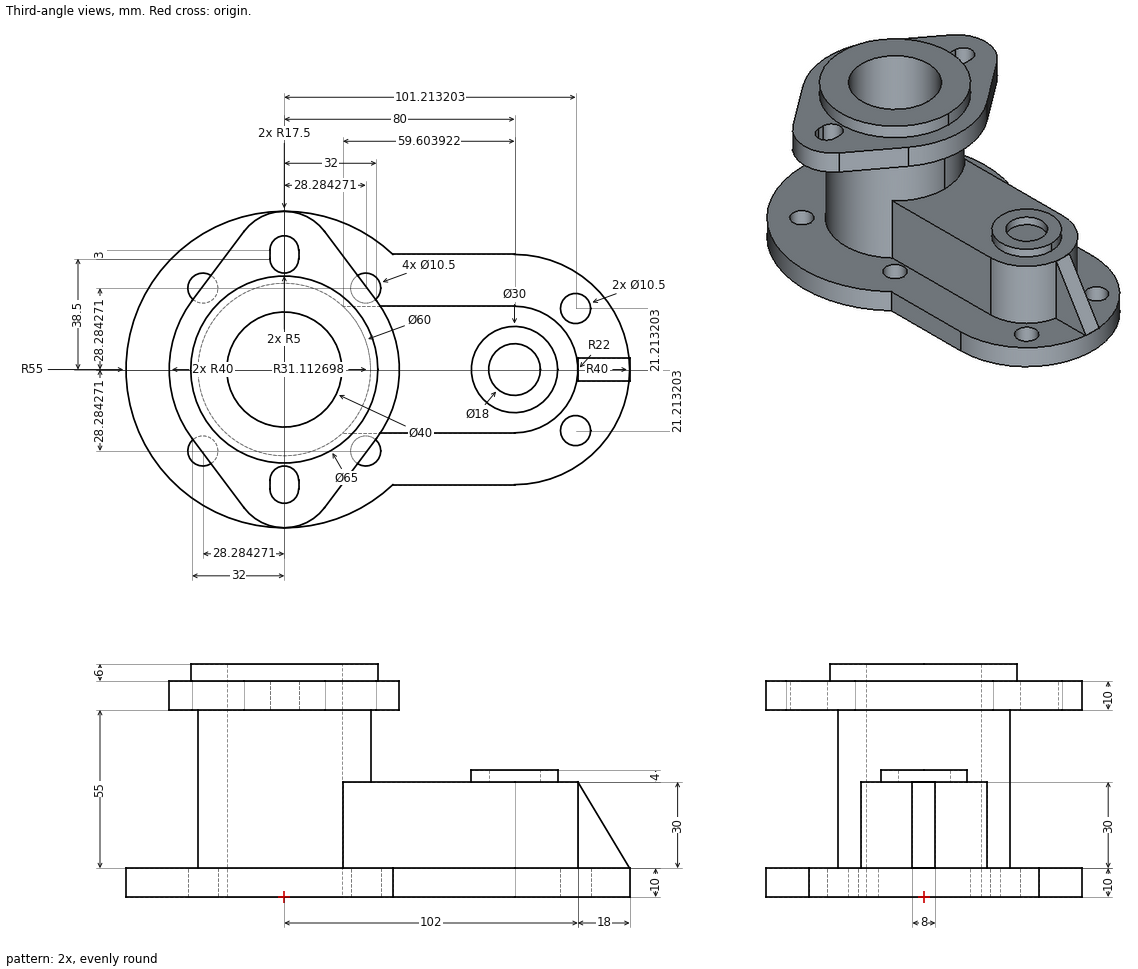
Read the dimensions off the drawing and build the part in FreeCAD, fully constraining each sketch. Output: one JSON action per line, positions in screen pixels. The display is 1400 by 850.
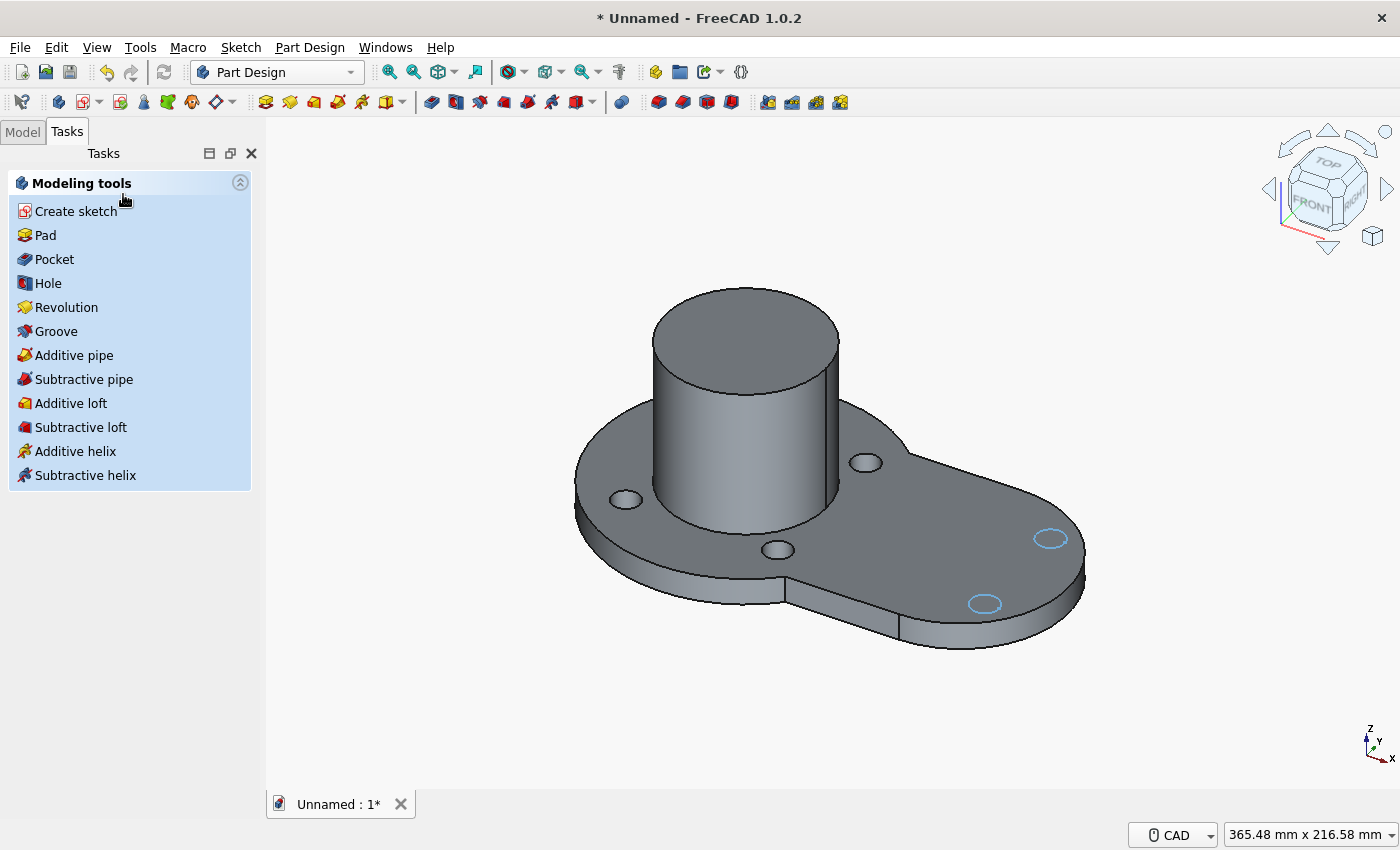
{"action": "left_click", "coordinate": [432, 102]}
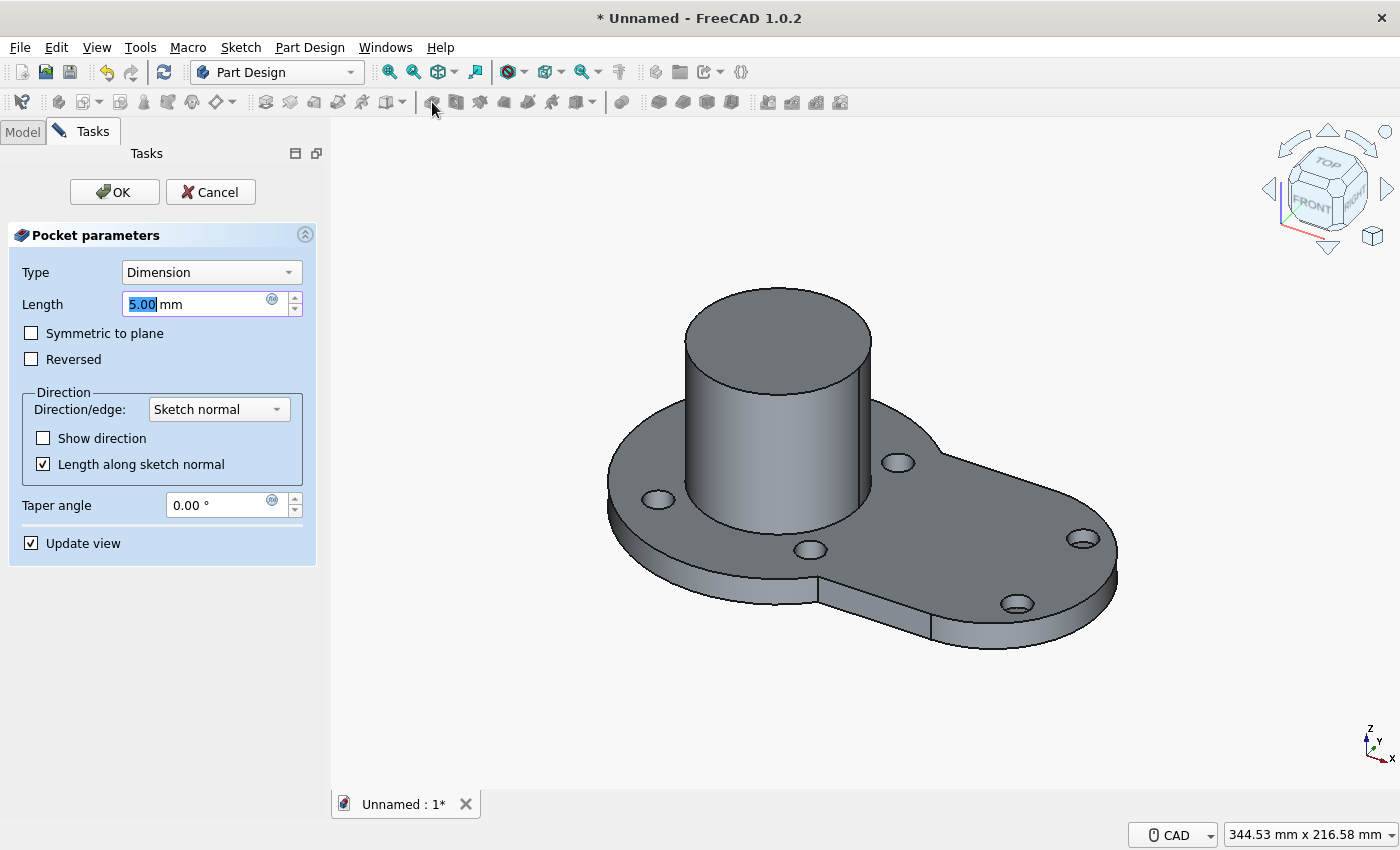
{"action": "left_click", "coordinate": [212, 272]}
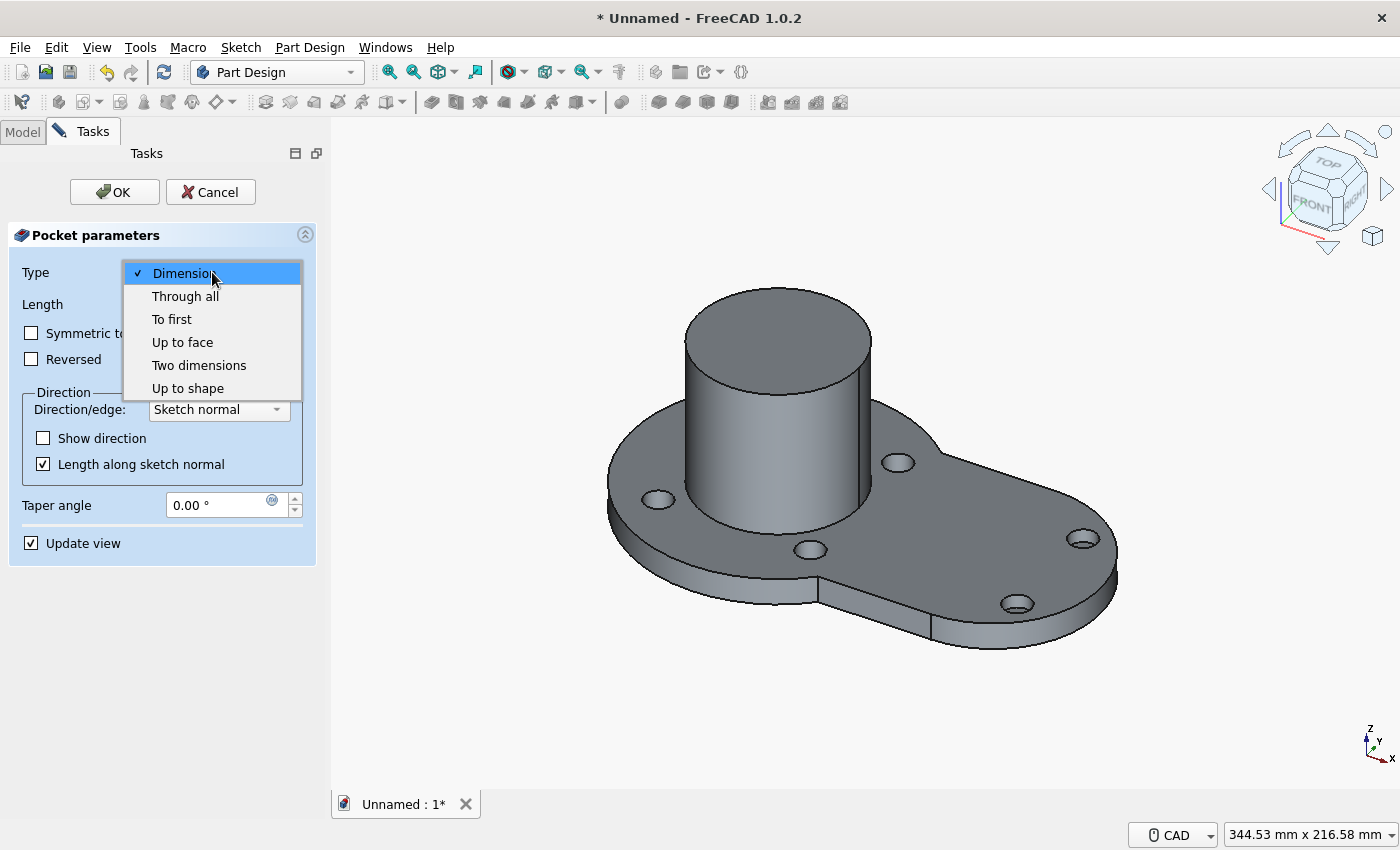
{"action": "left_click", "coordinate": [212, 296]}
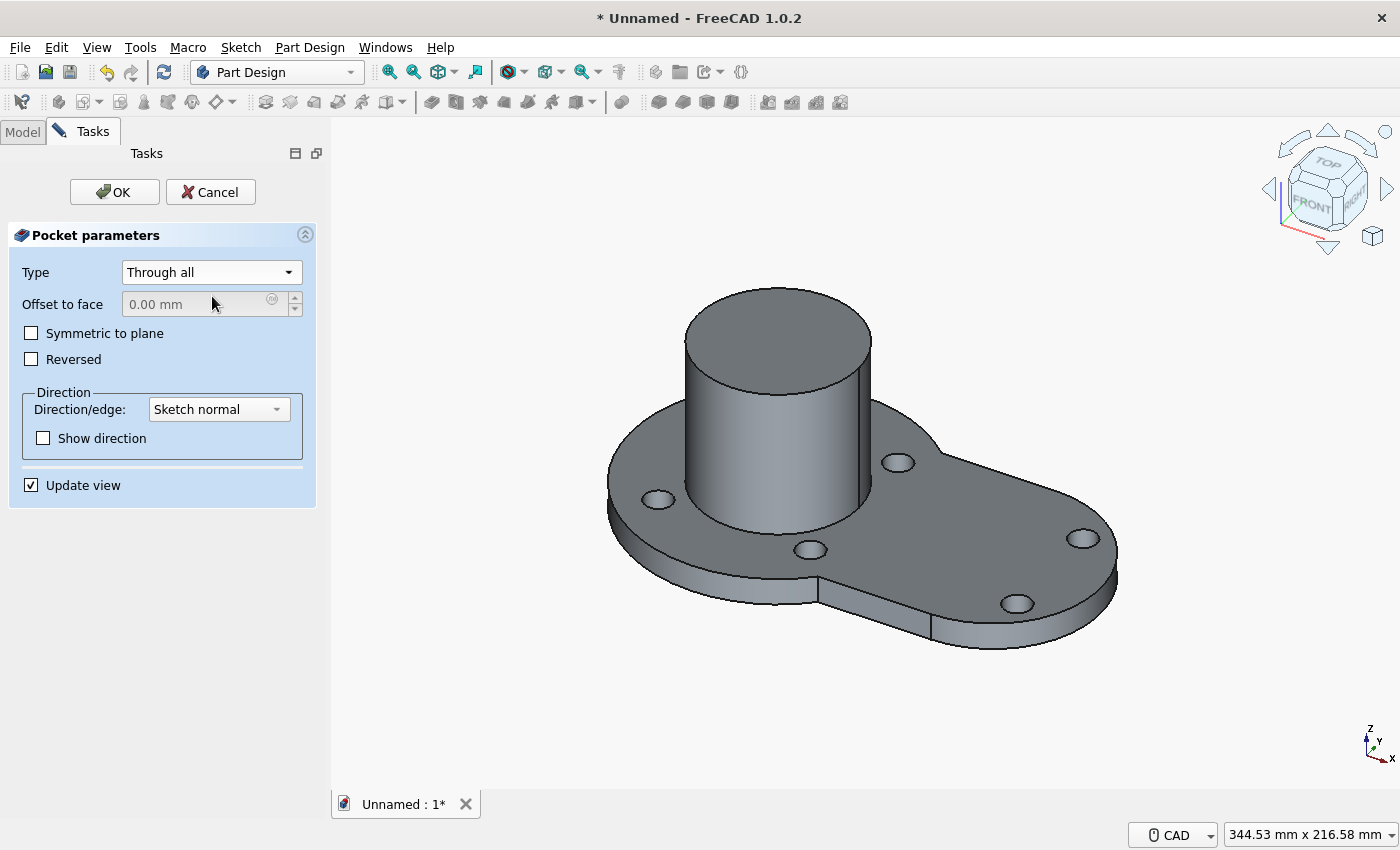
{"action": "left_click", "coordinate": [115, 192]}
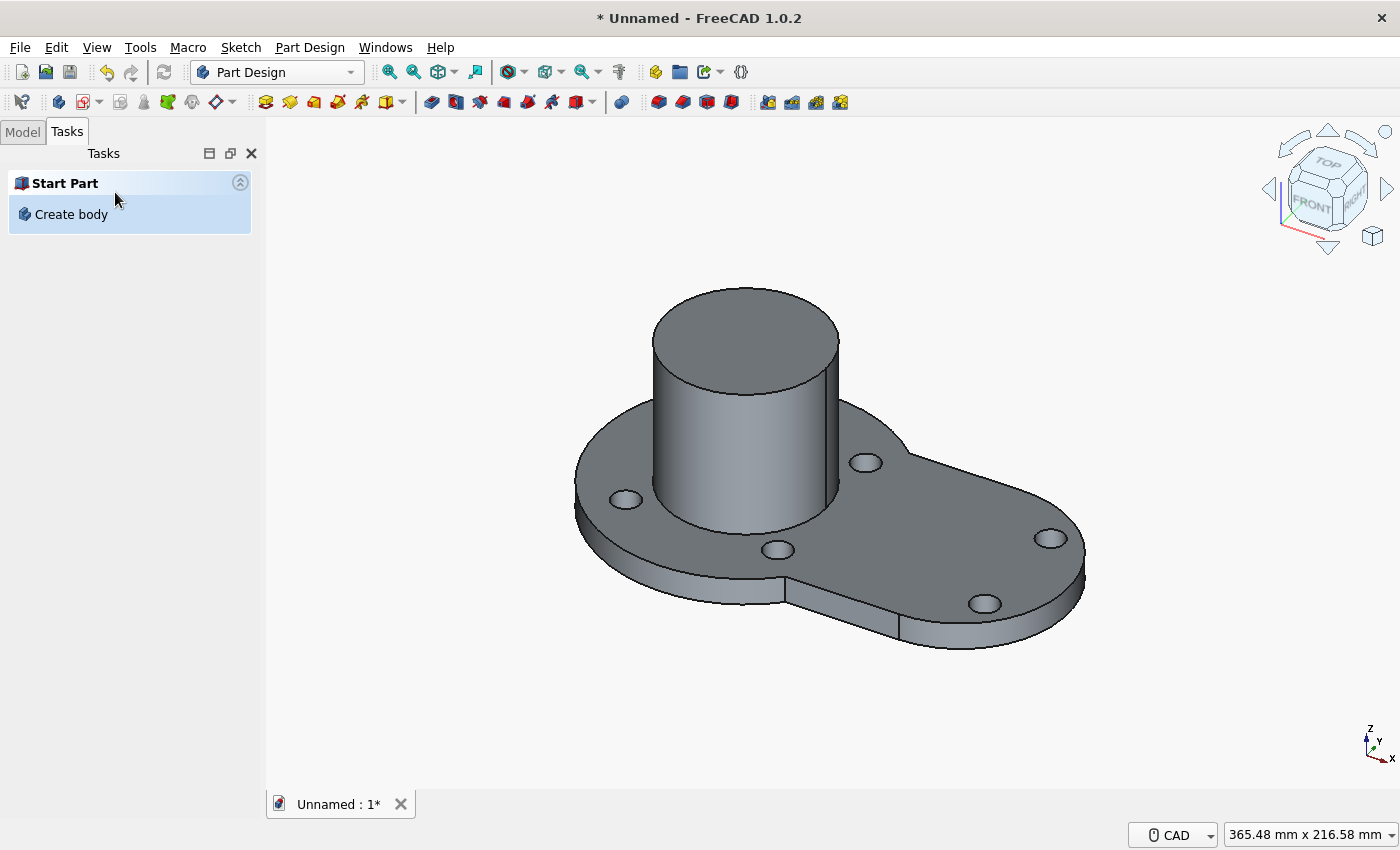
{"action": "left_click", "coordinate": [900, 531]}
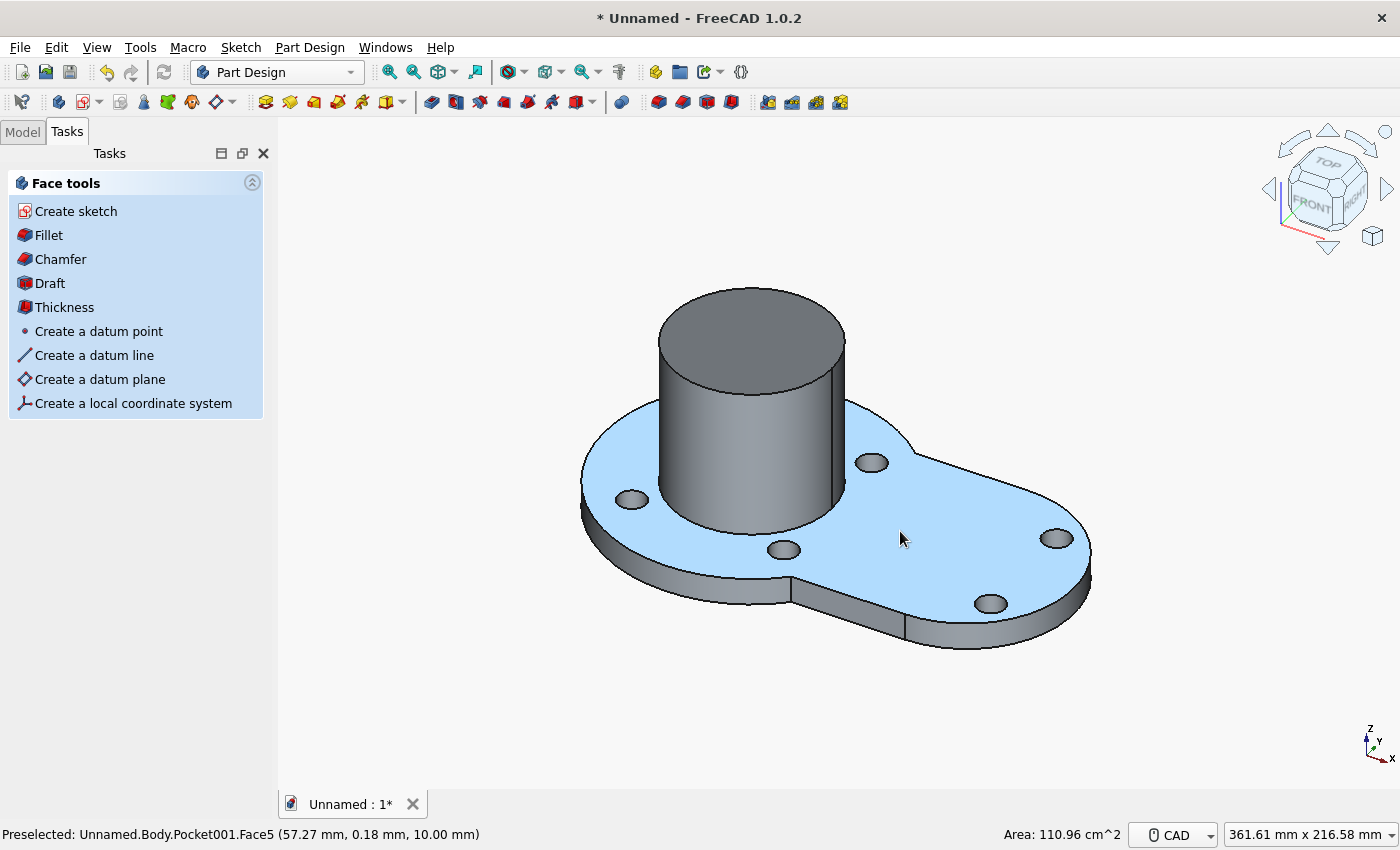
{"action": "left_click", "coordinate": [84, 102]}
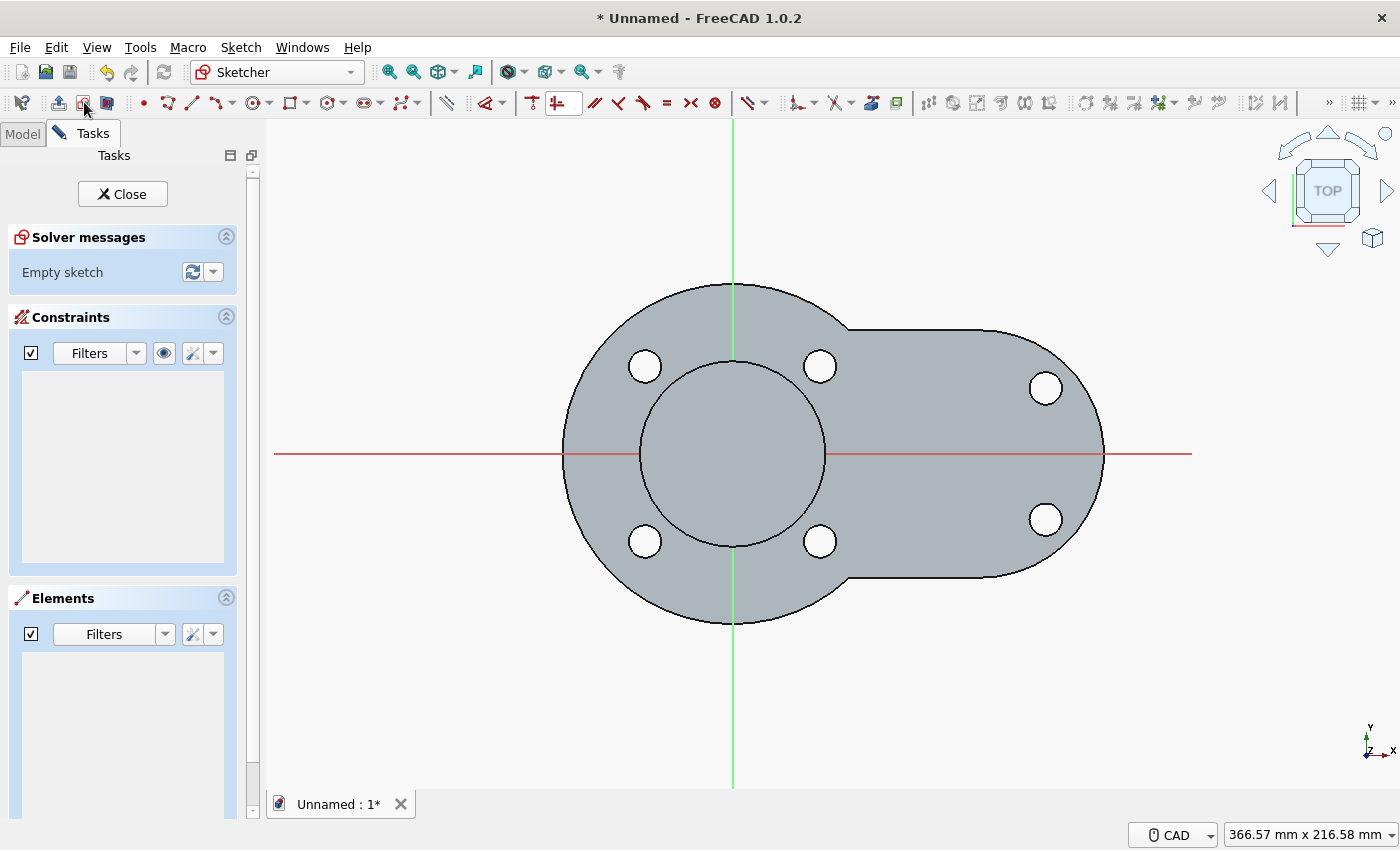
{"action": "scroll", "coordinate": [993, 454], "scroll_direction": "up", "scroll_amount": 4}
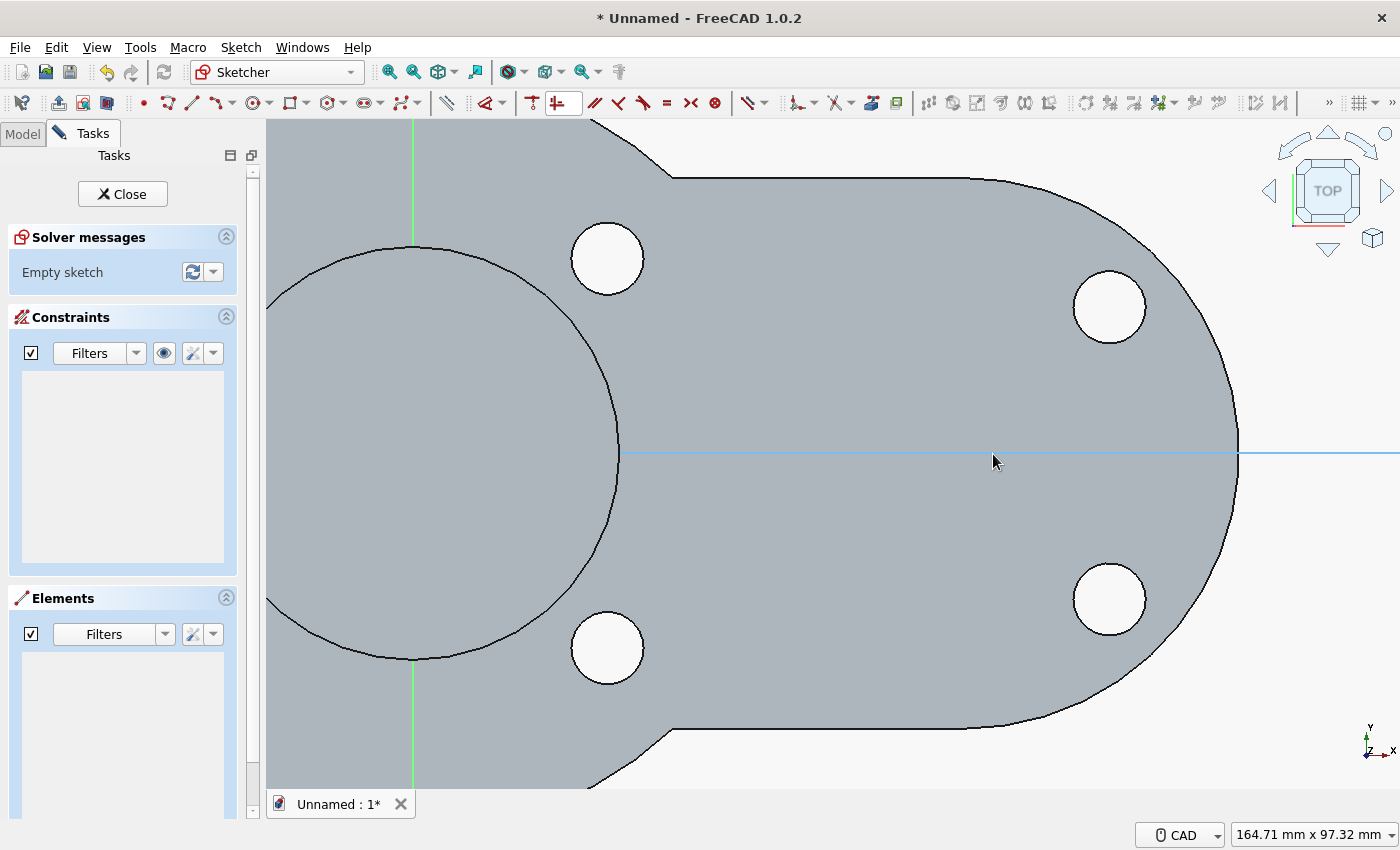
{"action": "key", "text": "g l"}